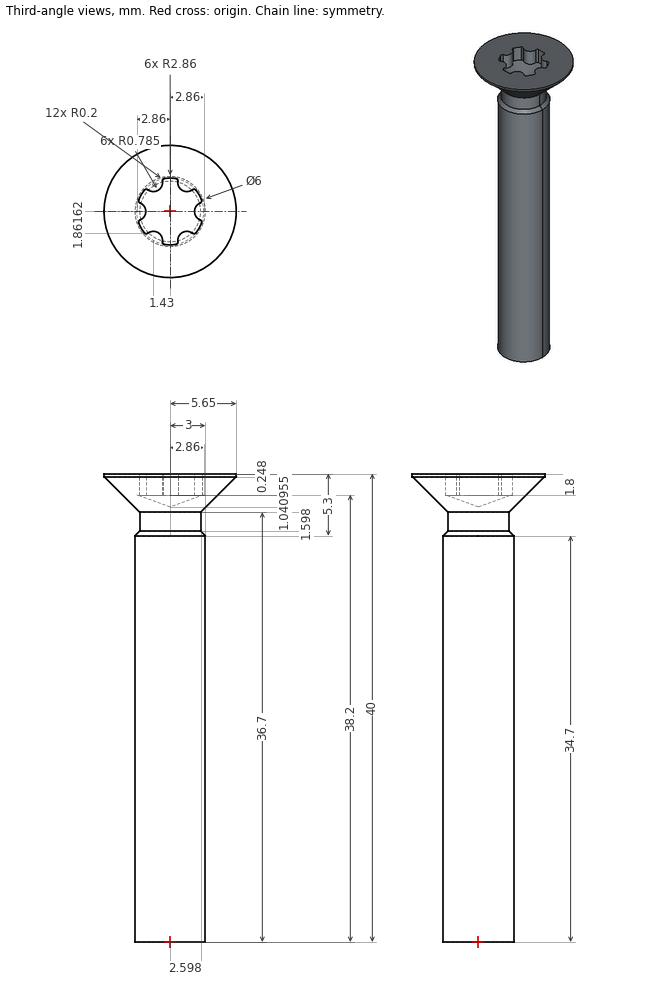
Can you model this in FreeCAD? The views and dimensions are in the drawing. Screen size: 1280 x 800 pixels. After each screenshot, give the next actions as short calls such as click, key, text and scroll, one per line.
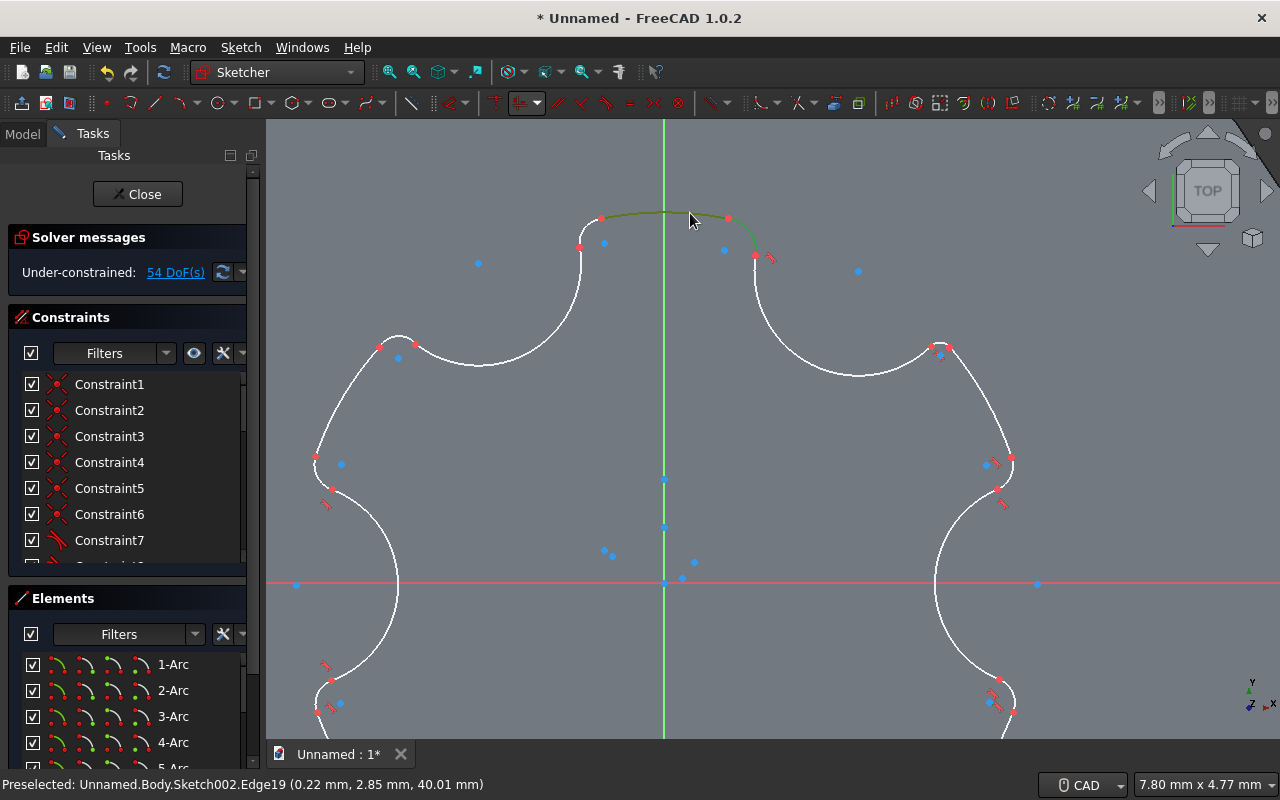
key(t)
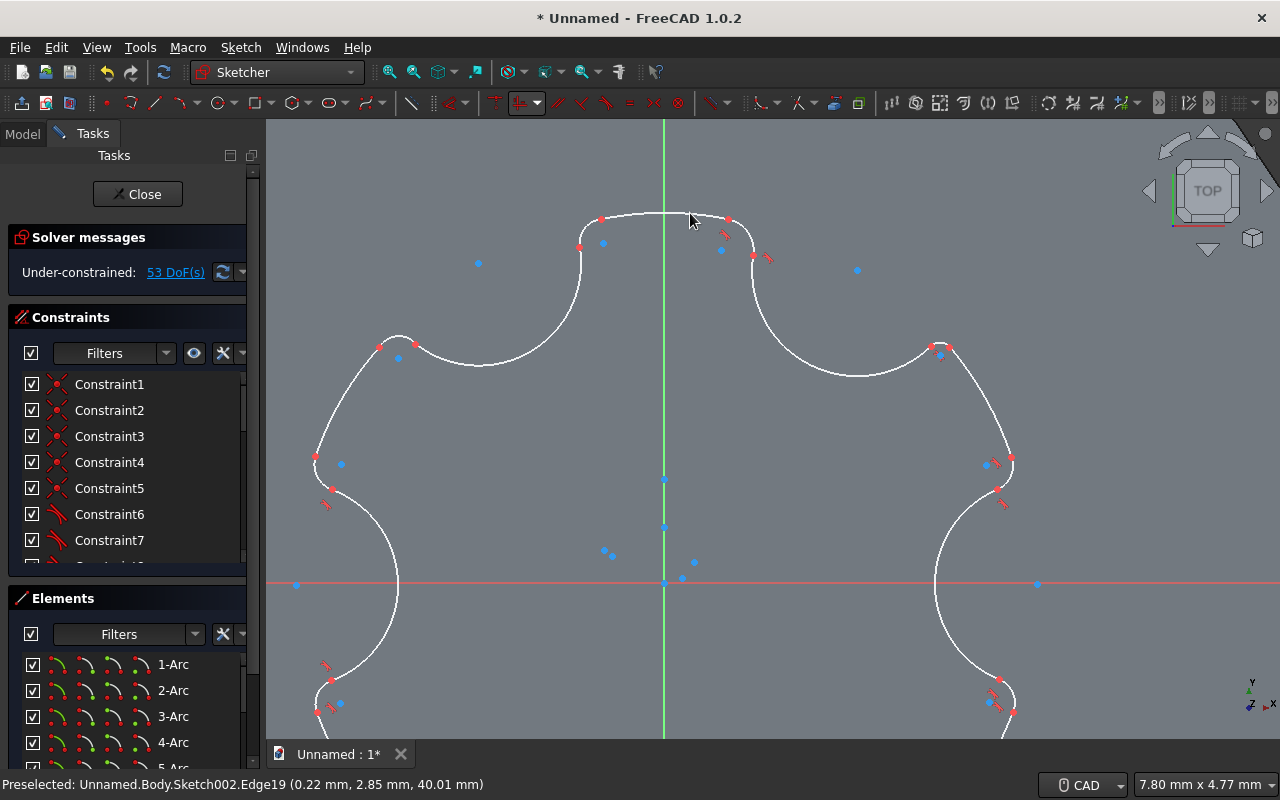
click(690, 214)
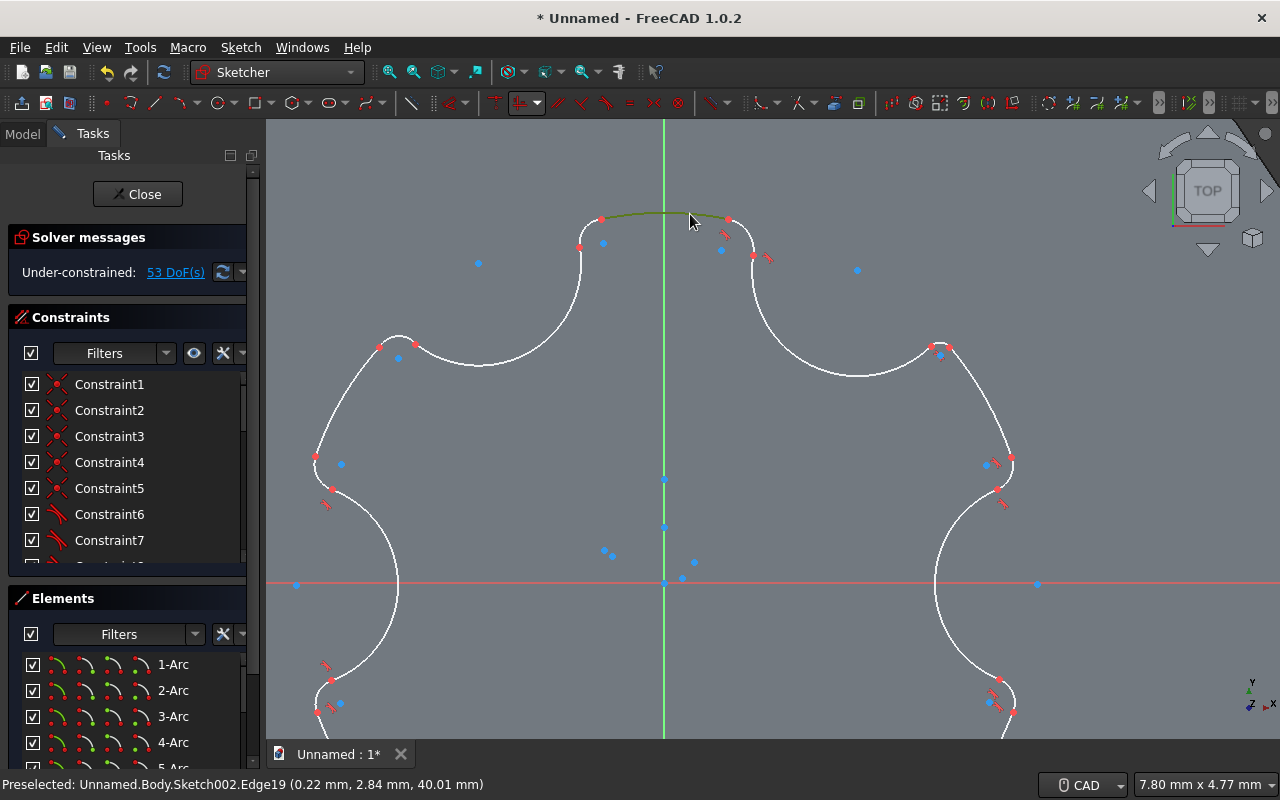
click(590, 223)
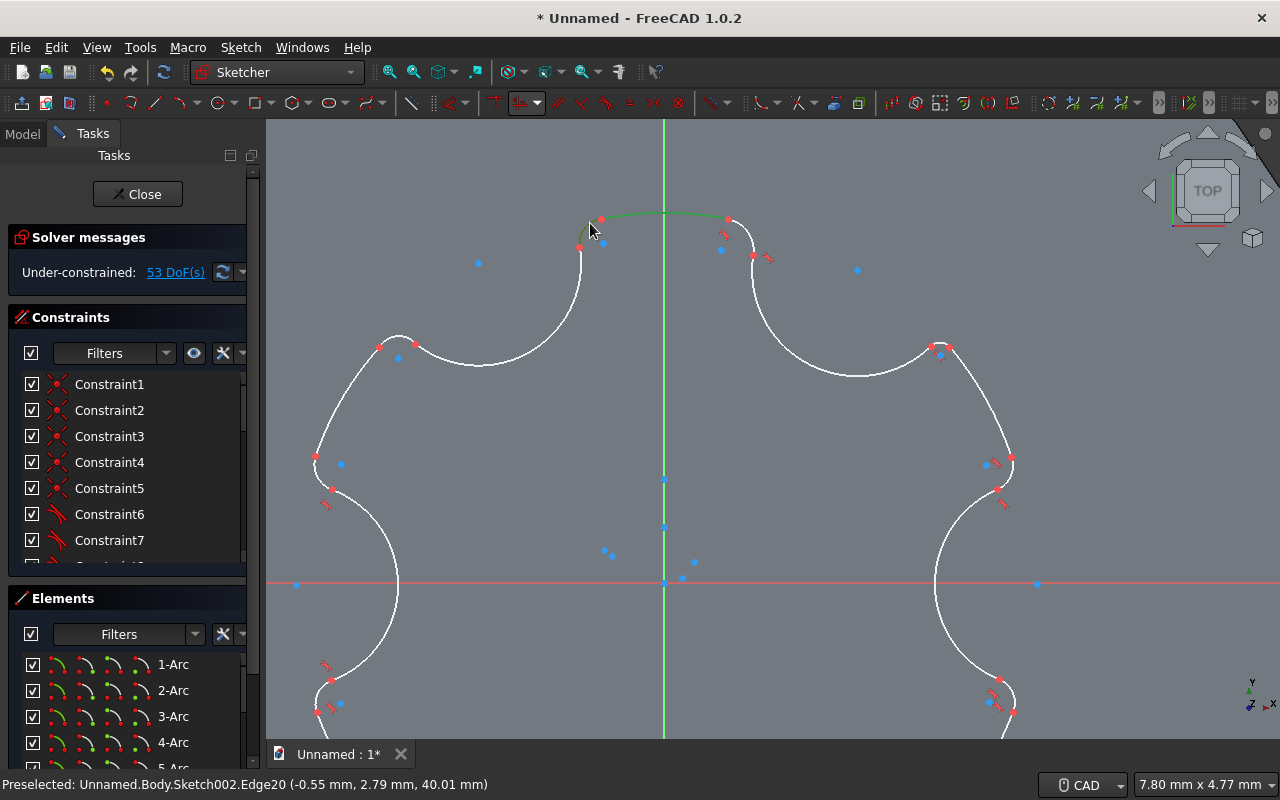
click(606, 104)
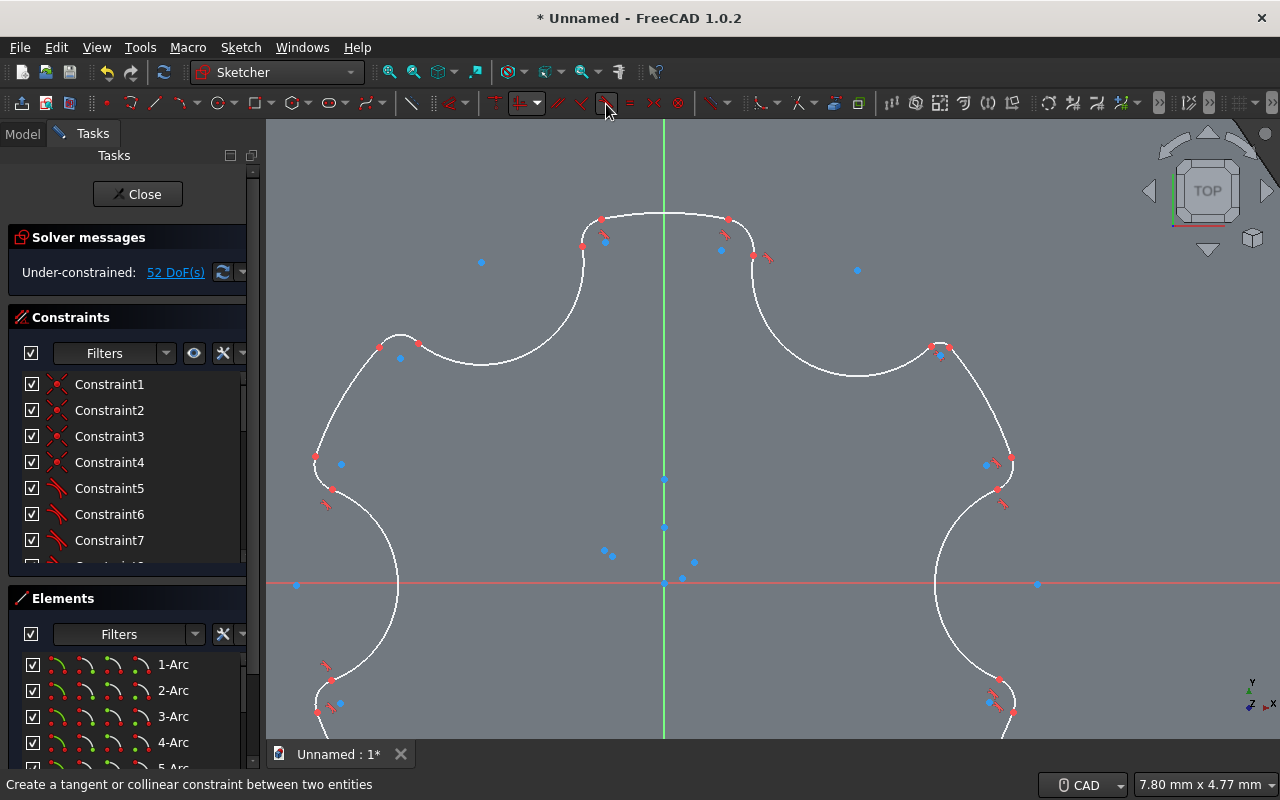
scroll(591, 224, up, 2)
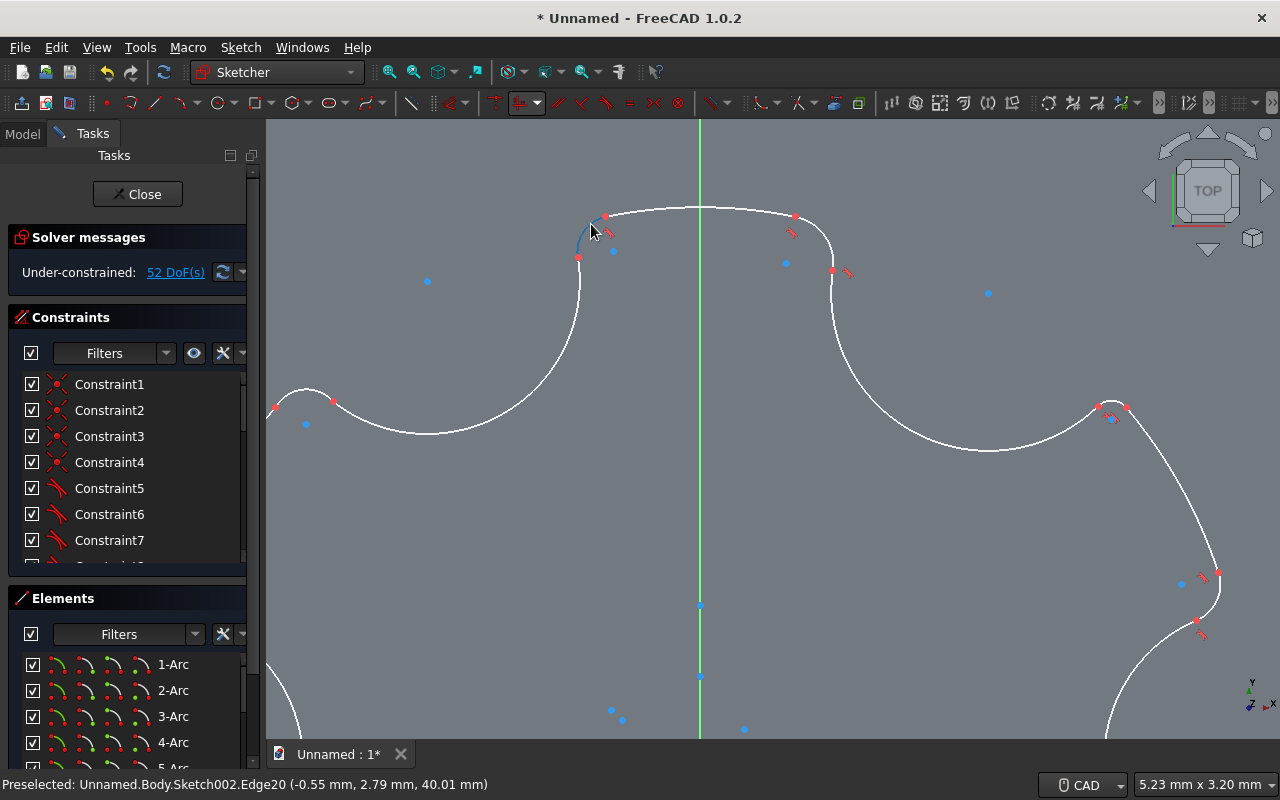
click(591, 224)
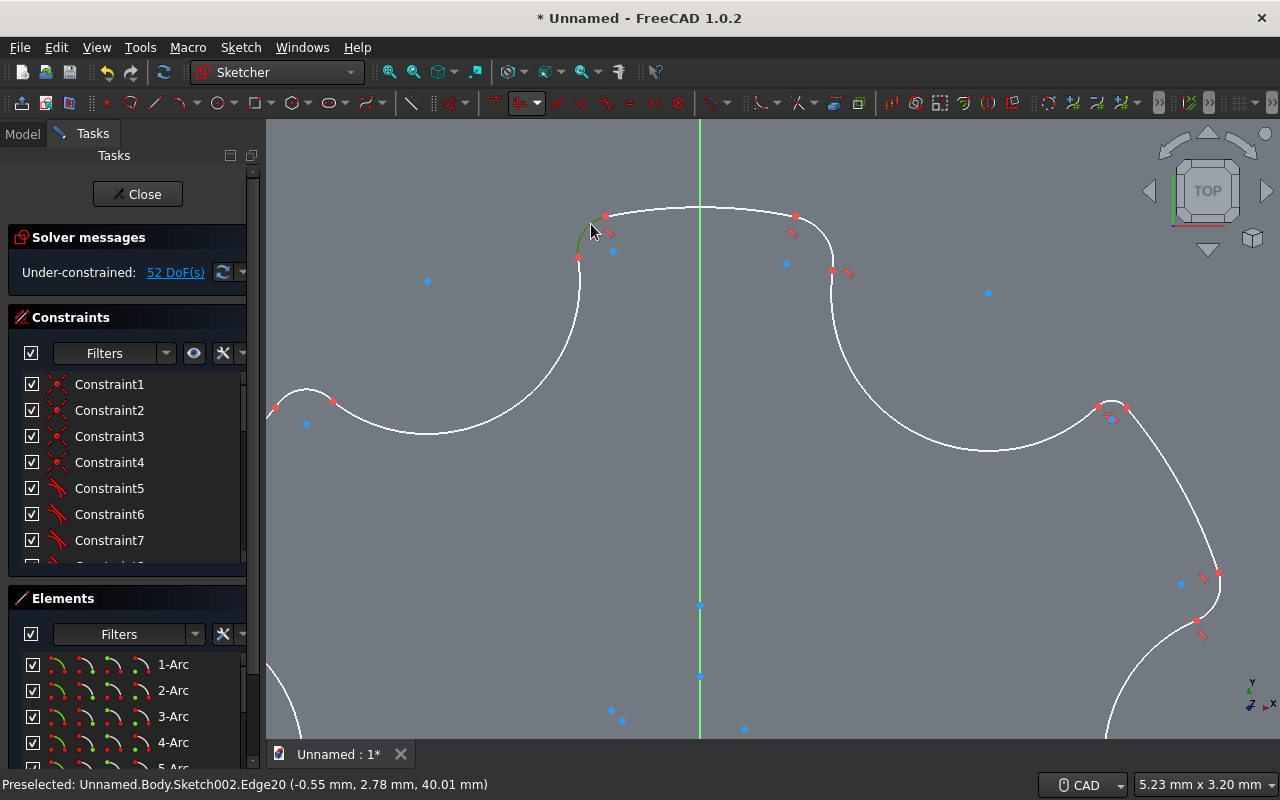
click(436, 434)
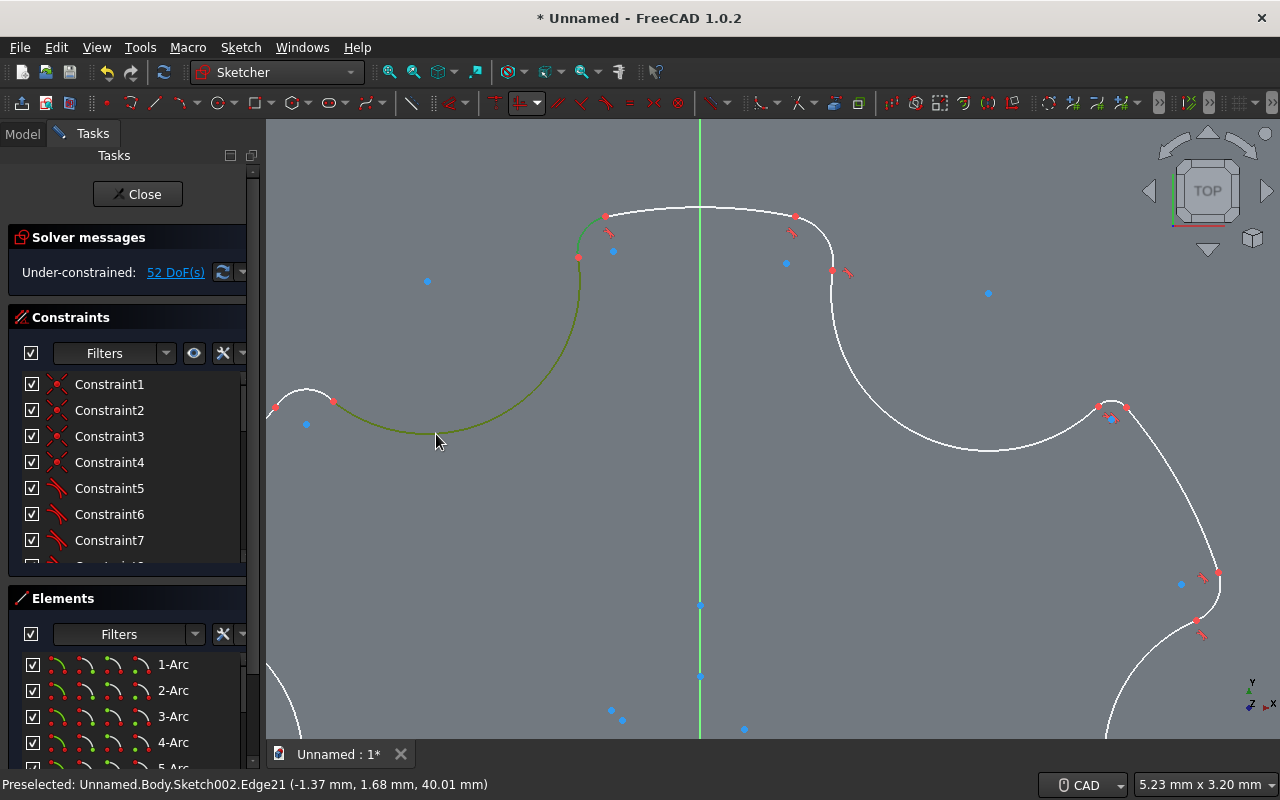
click(606, 104)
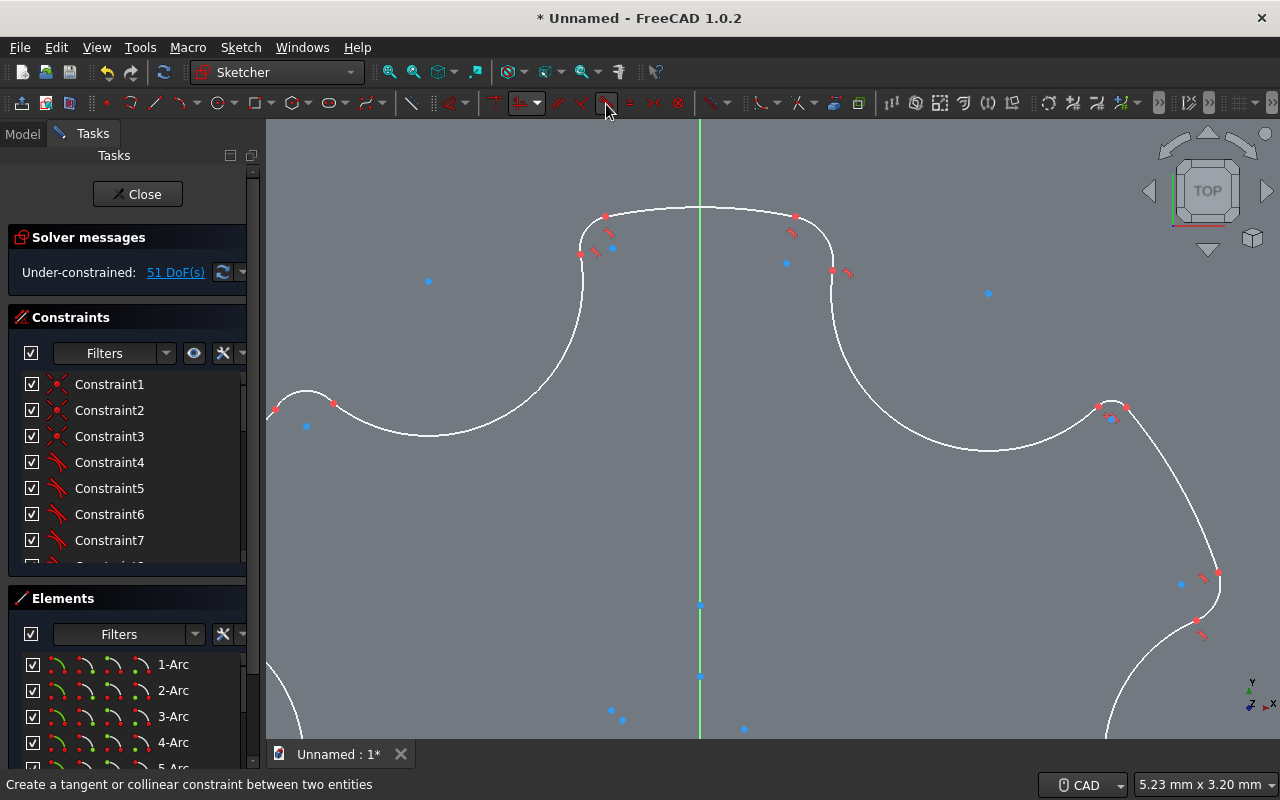
click(438, 436)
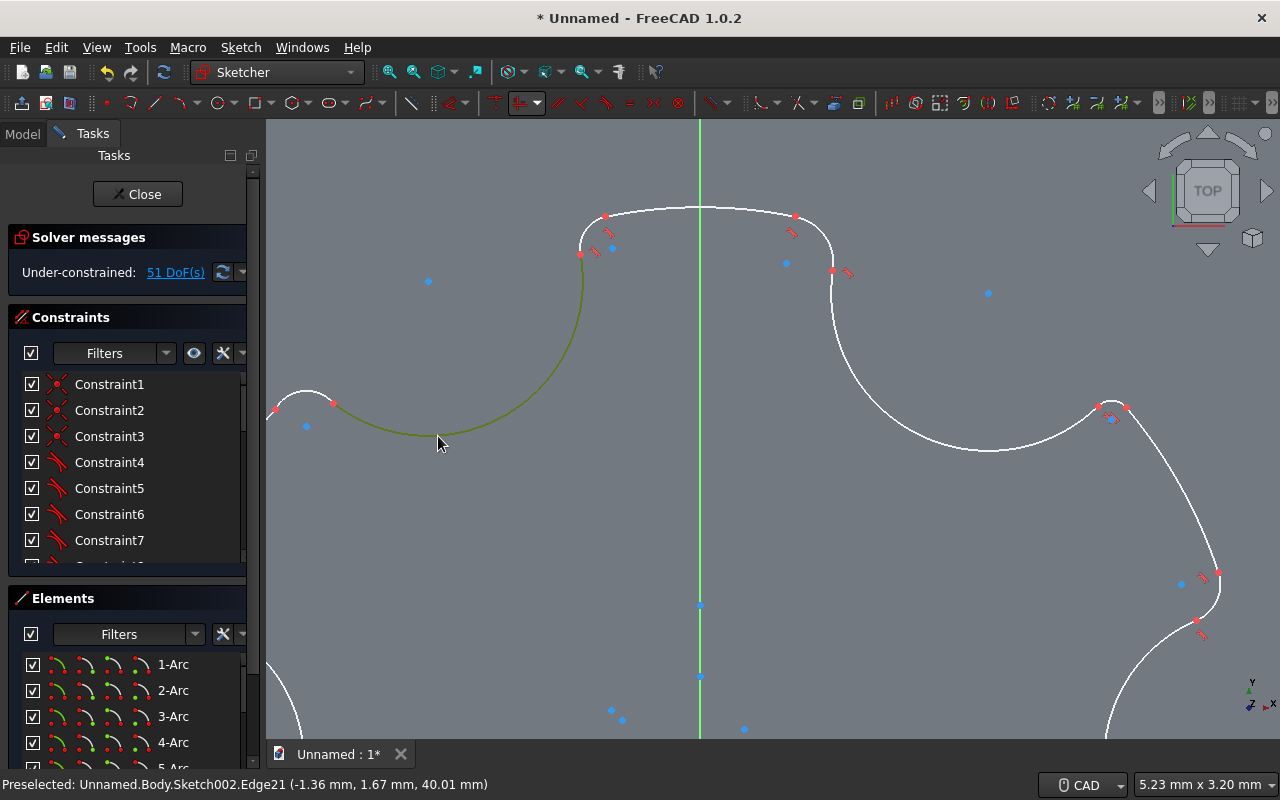
click(317, 392)